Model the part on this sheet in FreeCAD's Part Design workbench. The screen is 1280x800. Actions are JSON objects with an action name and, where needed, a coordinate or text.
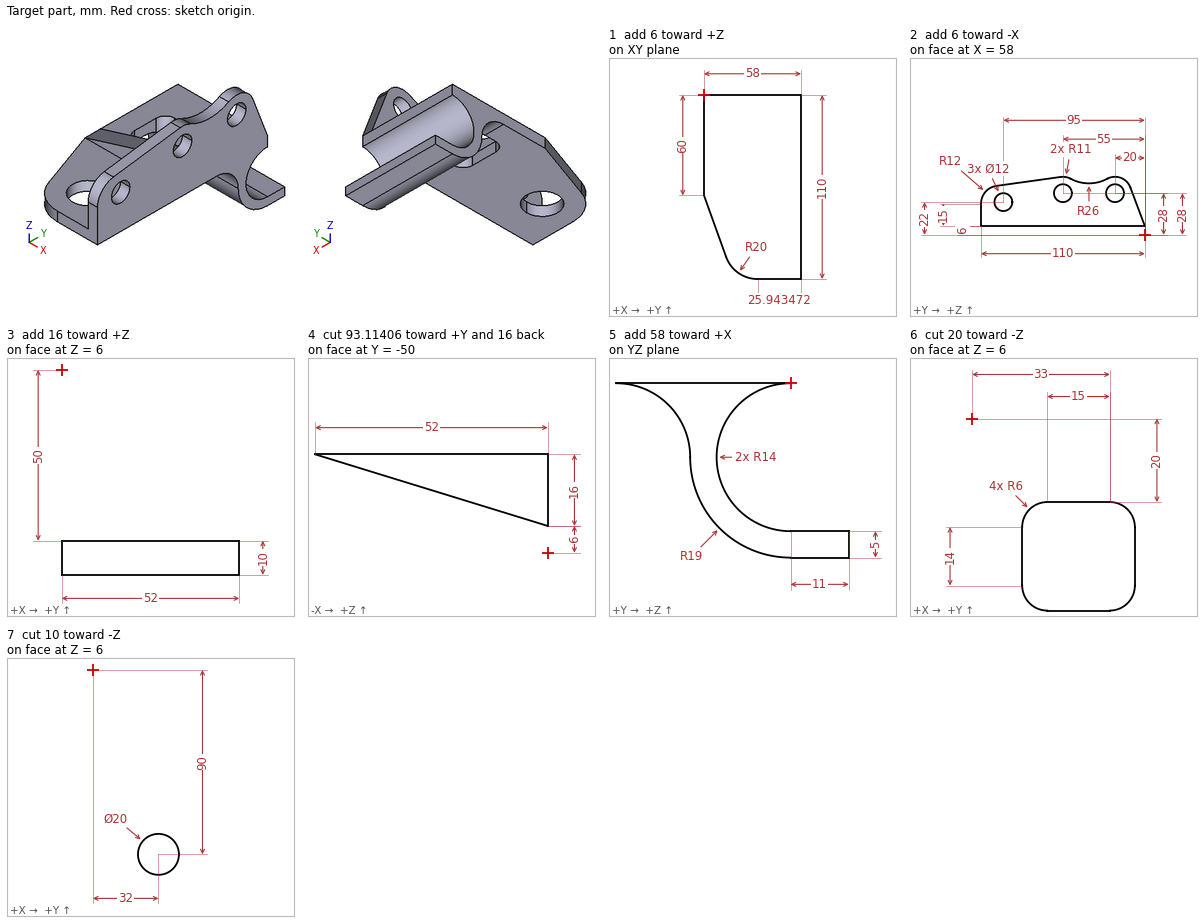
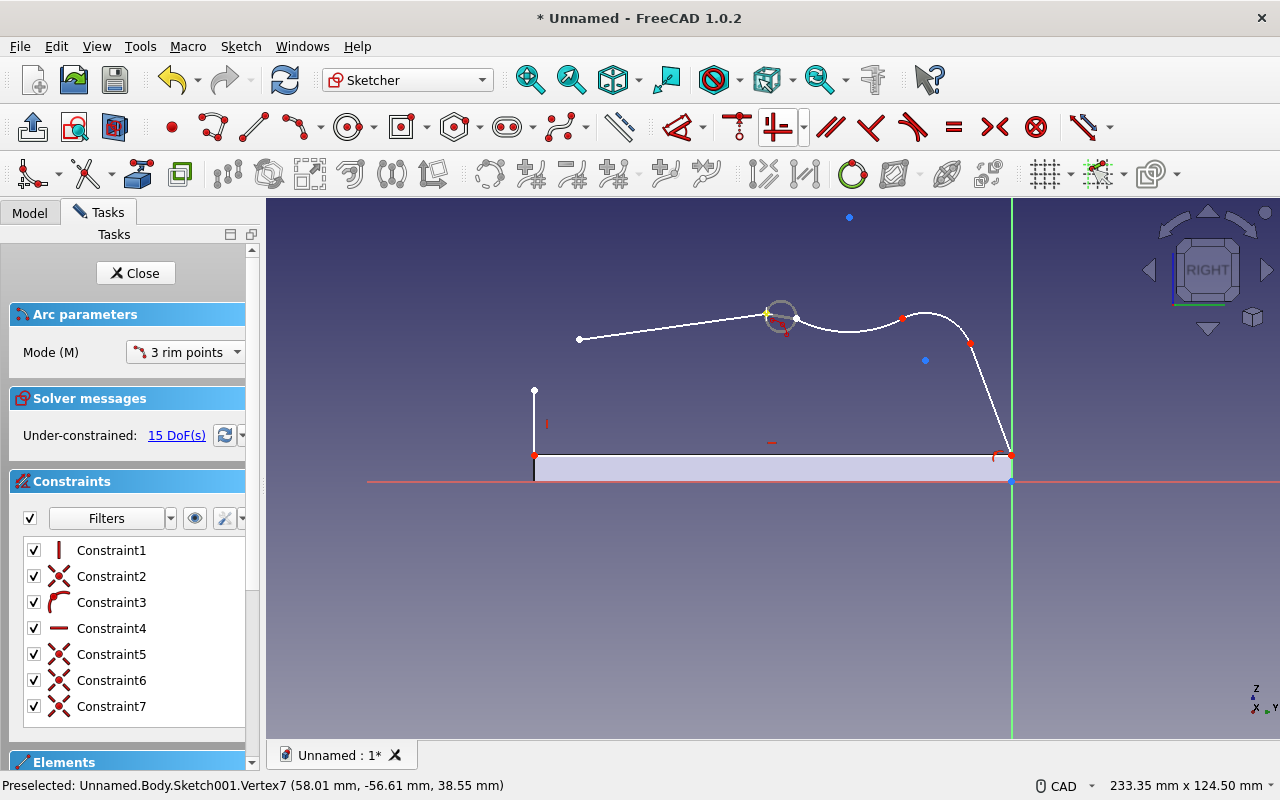
{"action": "scroll", "coordinate": [781, 313], "scroll_direction": "up", "scroll_amount": 10}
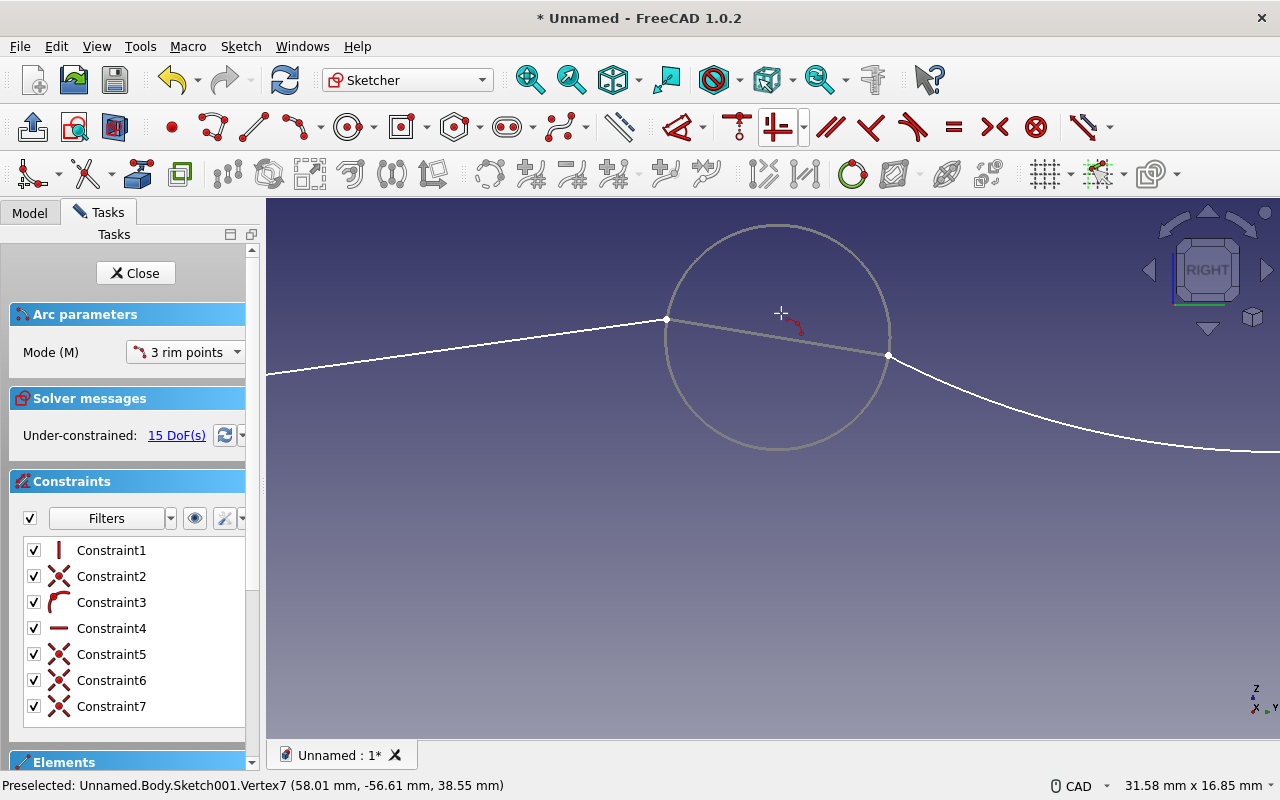
{"action": "left_click", "coordinate": [781, 310]}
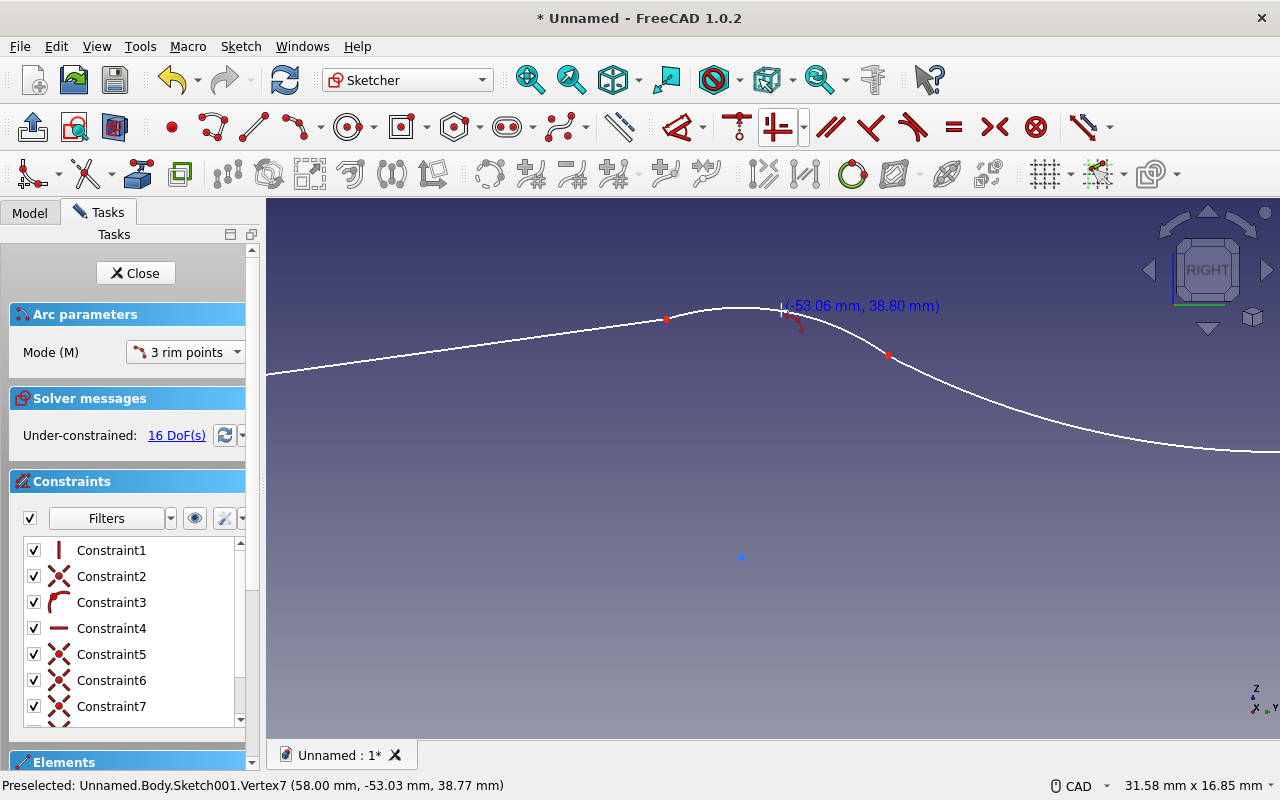
{"action": "scroll", "coordinate": [702, 377], "scroll_direction": "down", "scroll_amount": 9}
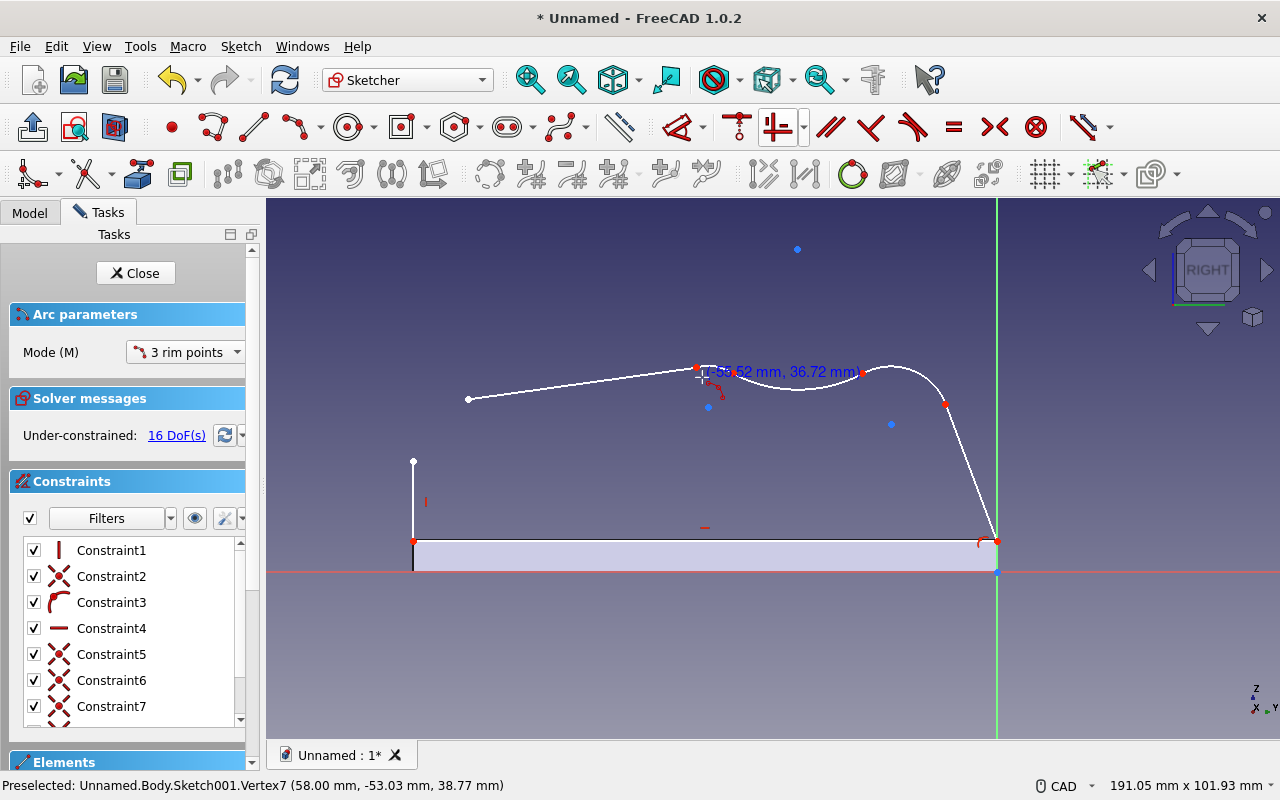
{"action": "left_click", "coordinate": [468, 399]}
{"action": "left_click", "coordinate": [413, 462]}
{"action": "left_click", "coordinate": [429, 419]}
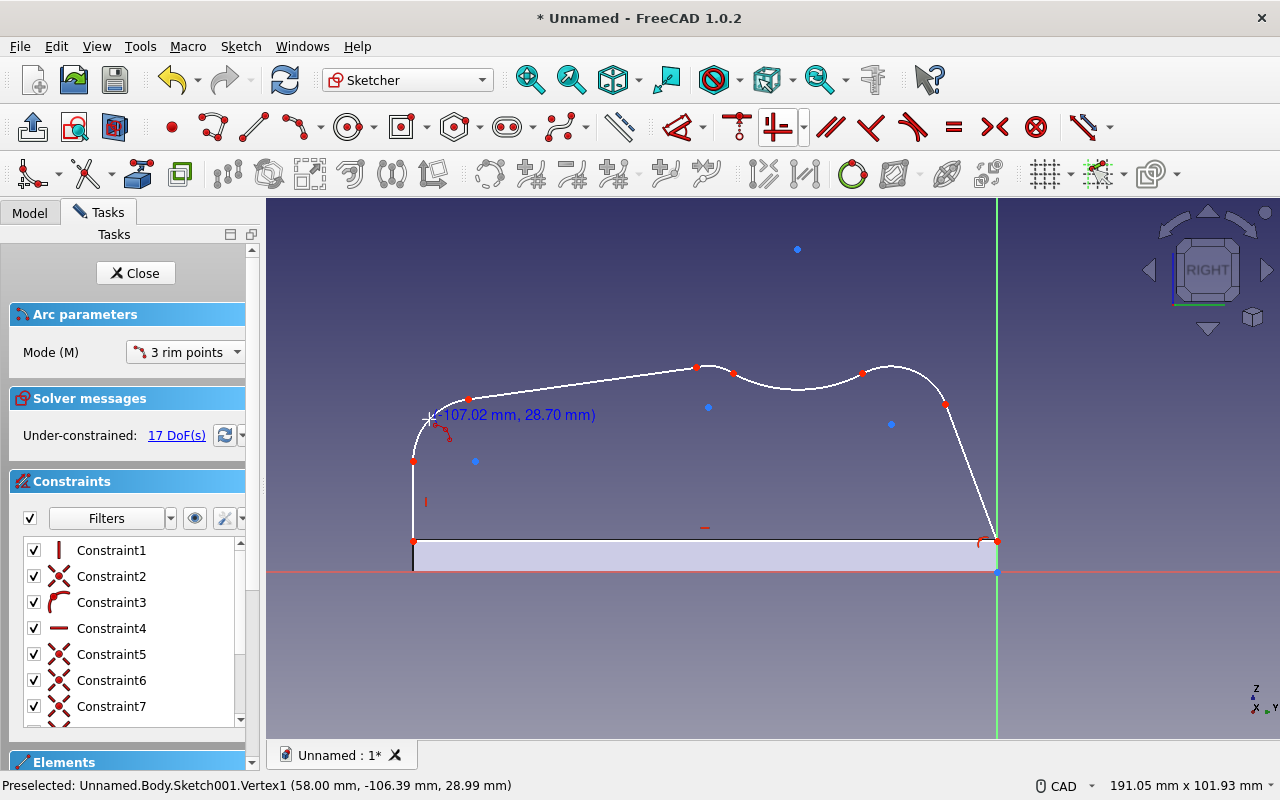
{"action": "key", "text": "g c"}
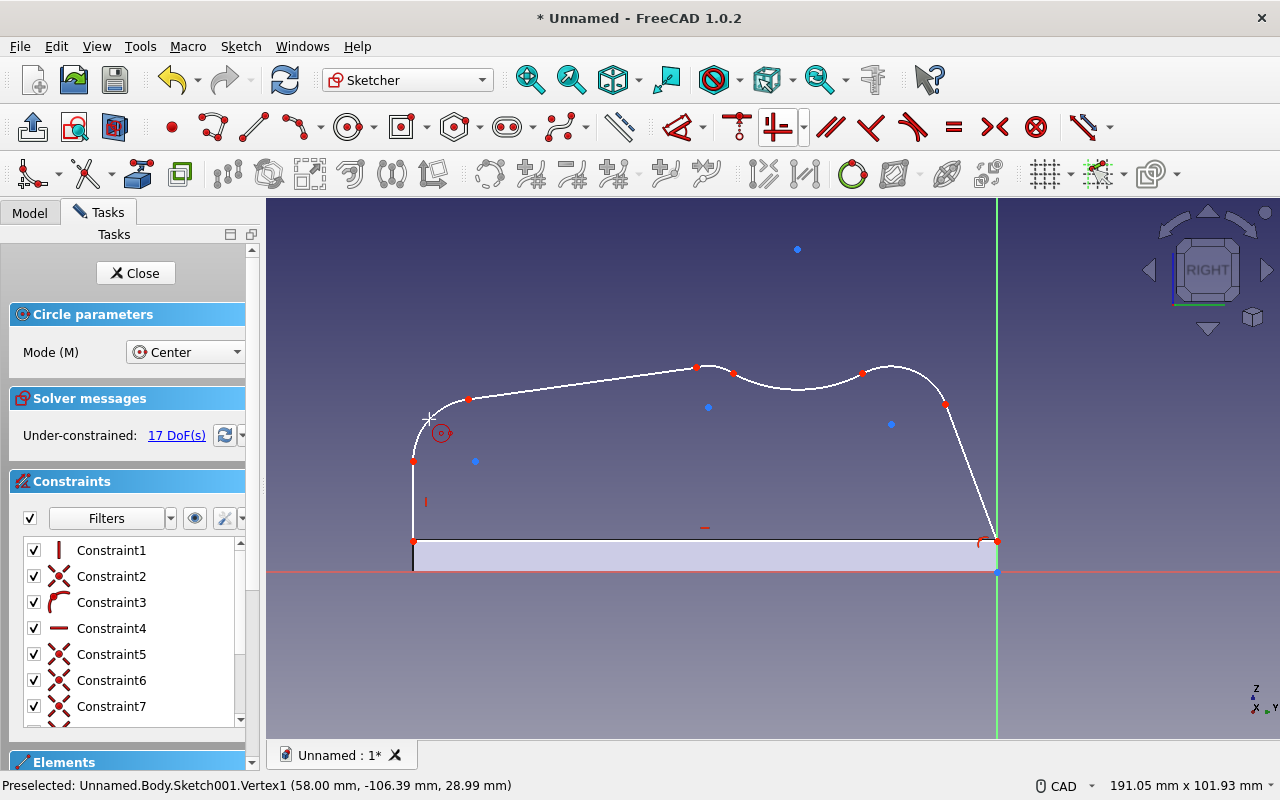
{"action": "left_click", "coordinate": [493, 456]}
{"action": "mouse_move", "coordinate": [515, 433]}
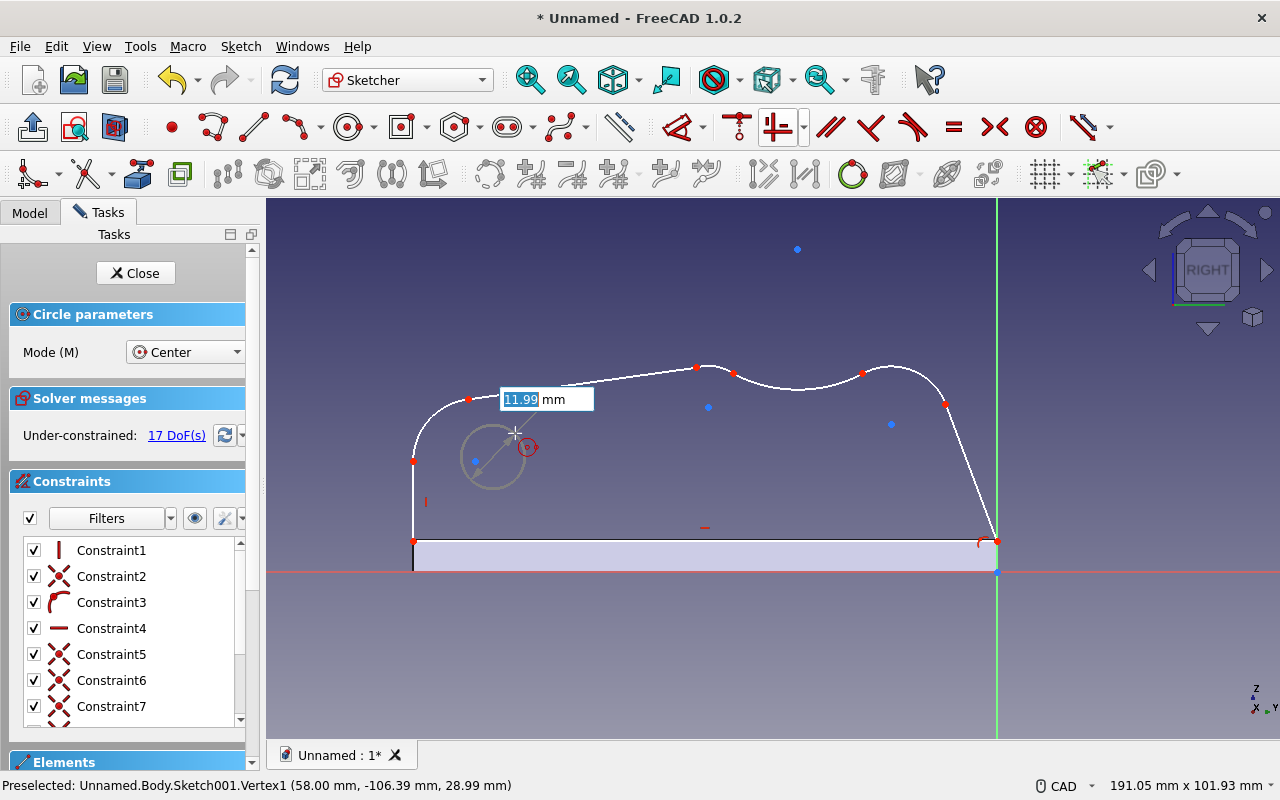
{"action": "type", "text": "12"}
{"action": "key", "text": "Return"}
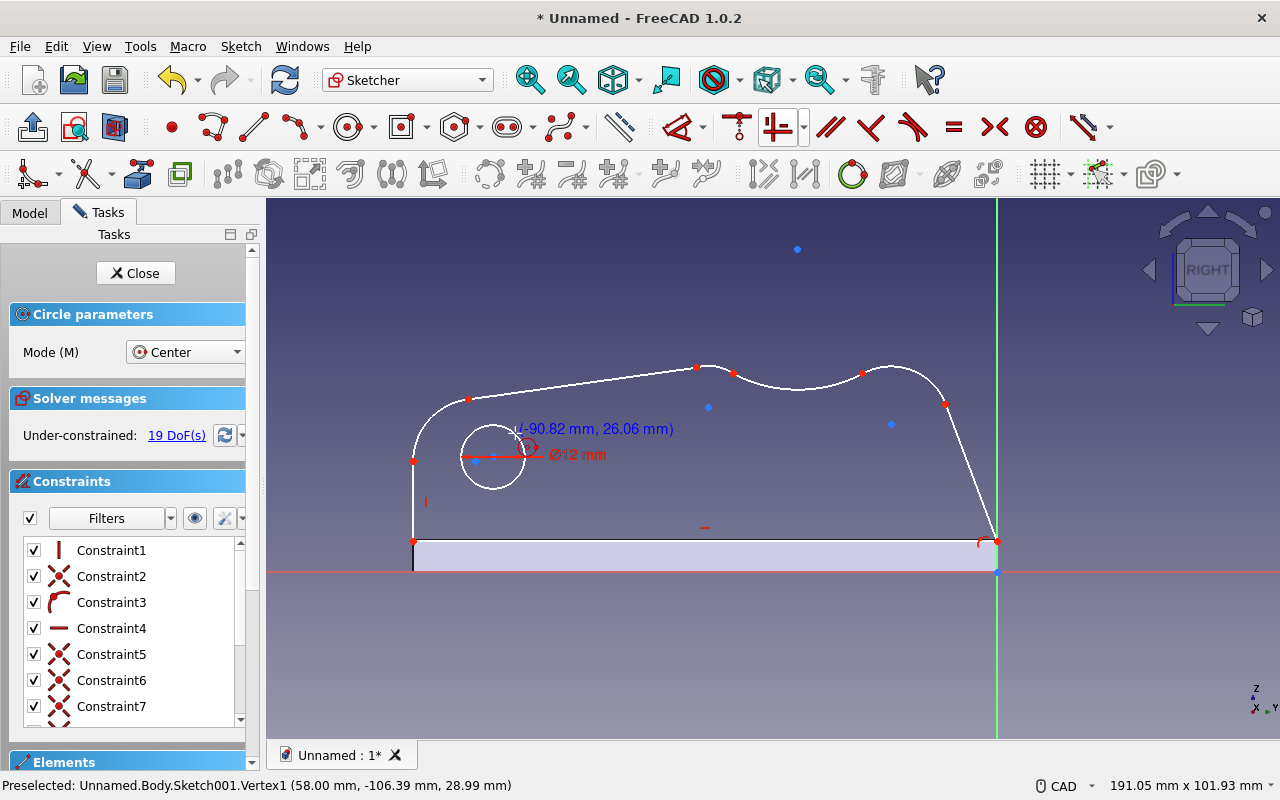
{"action": "left_click", "coordinate": [705, 424]}
{"action": "mouse_move", "coordinate": [728, 401]}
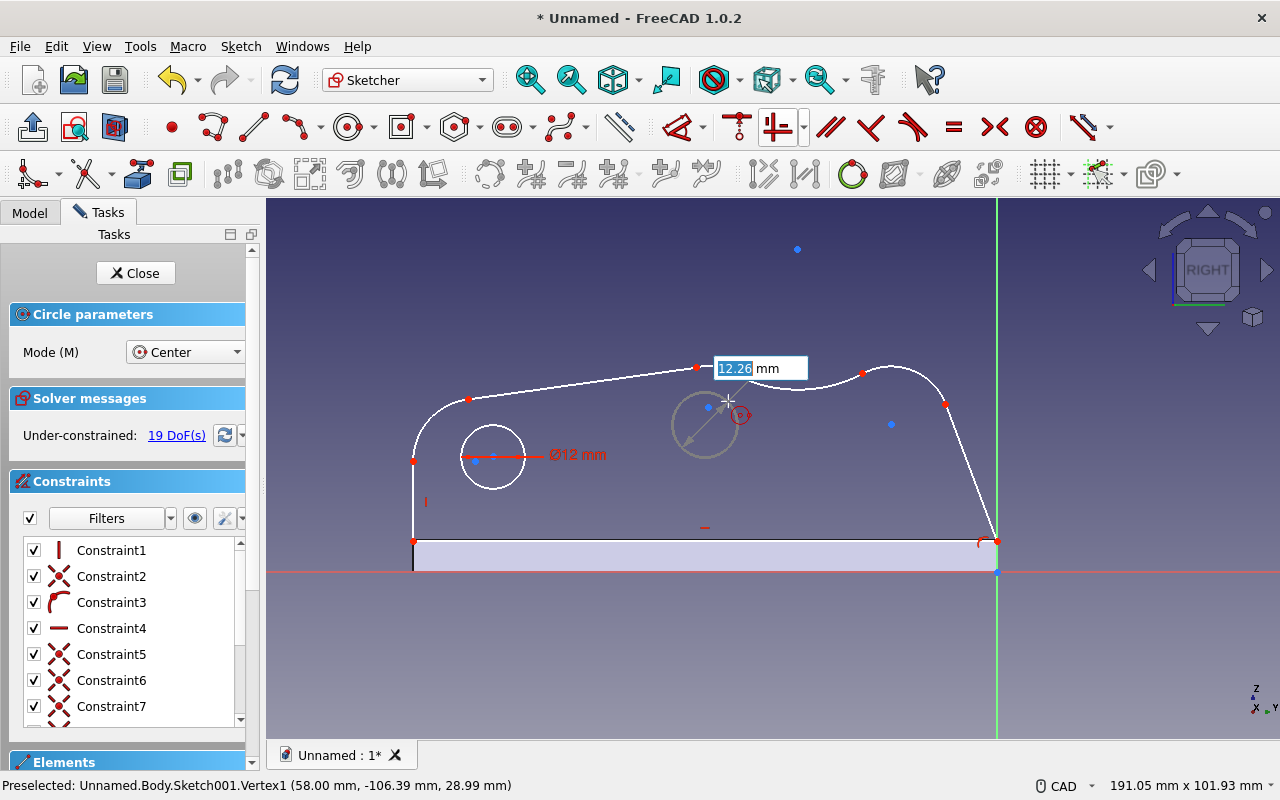
{"action": "type", "text": "12"}
{"action": "key", "text": "Return"}